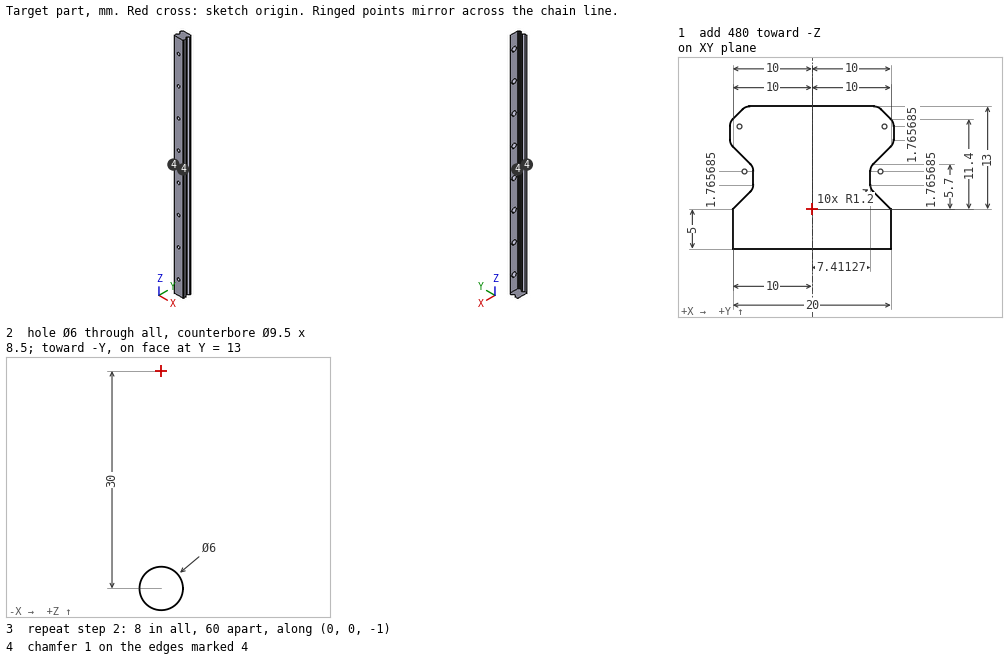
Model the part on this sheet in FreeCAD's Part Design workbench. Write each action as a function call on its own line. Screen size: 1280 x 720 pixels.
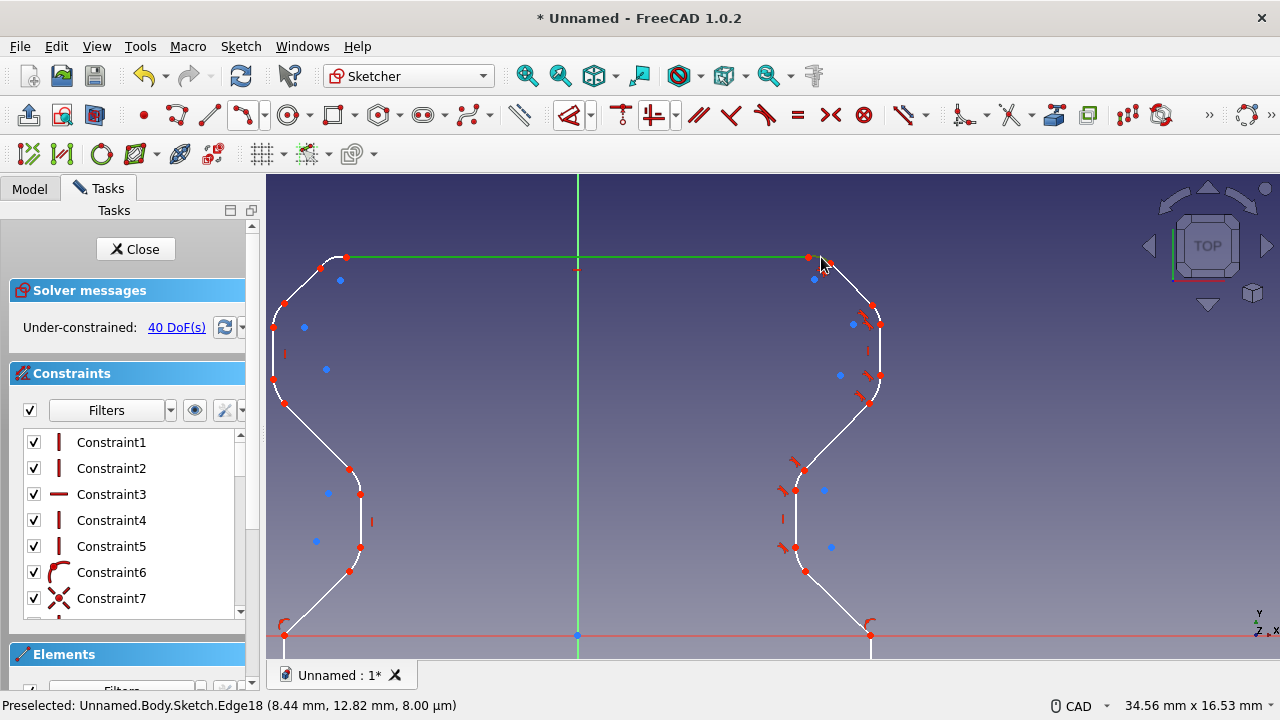
key(t)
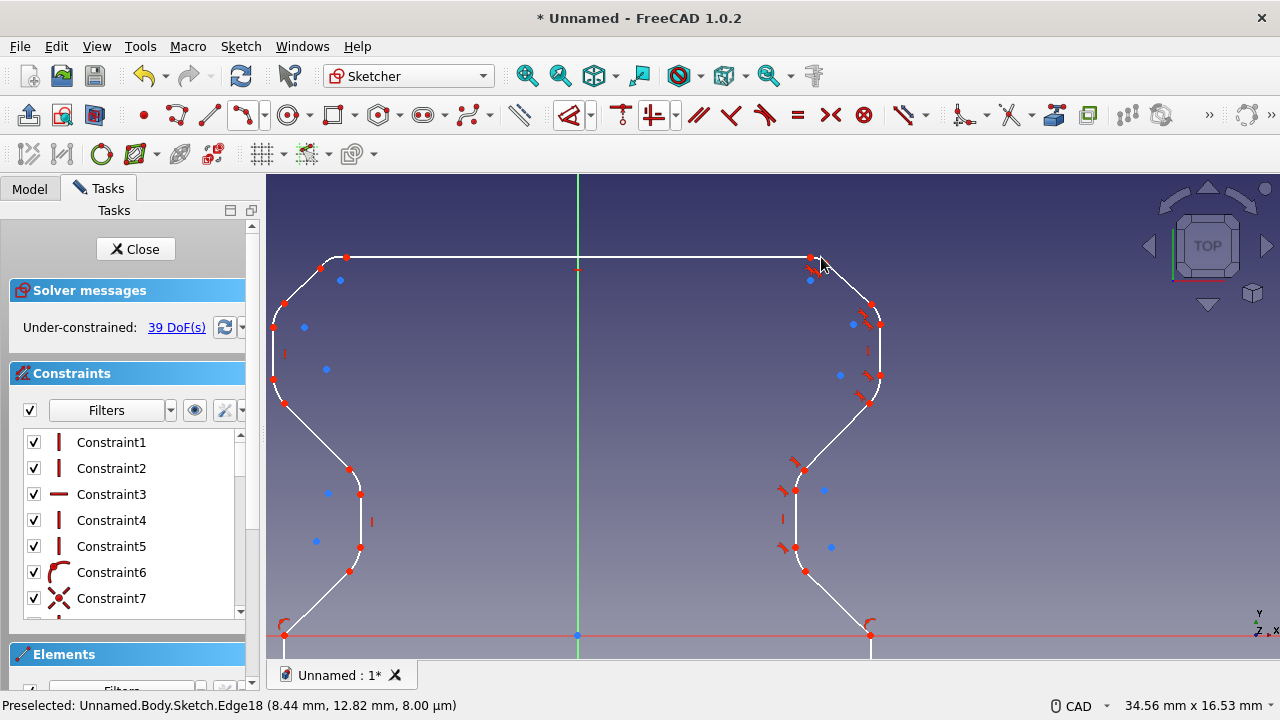
click(671, 257)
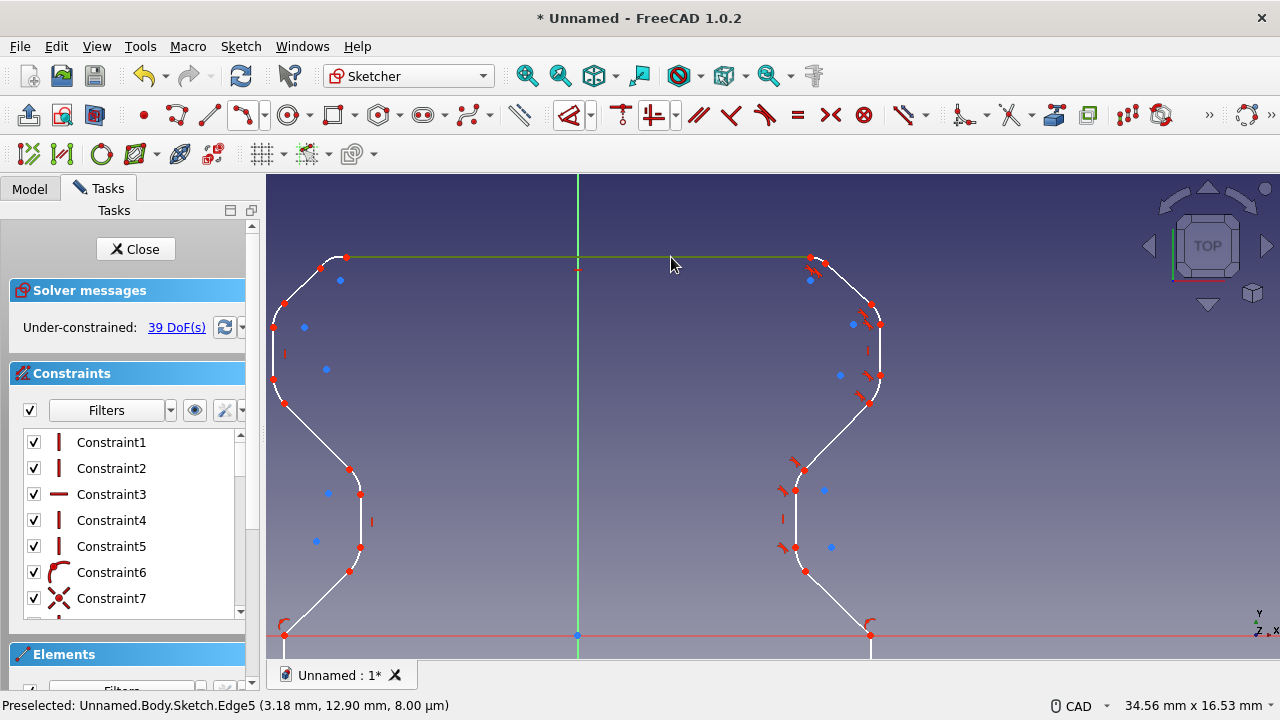
click(332, 258)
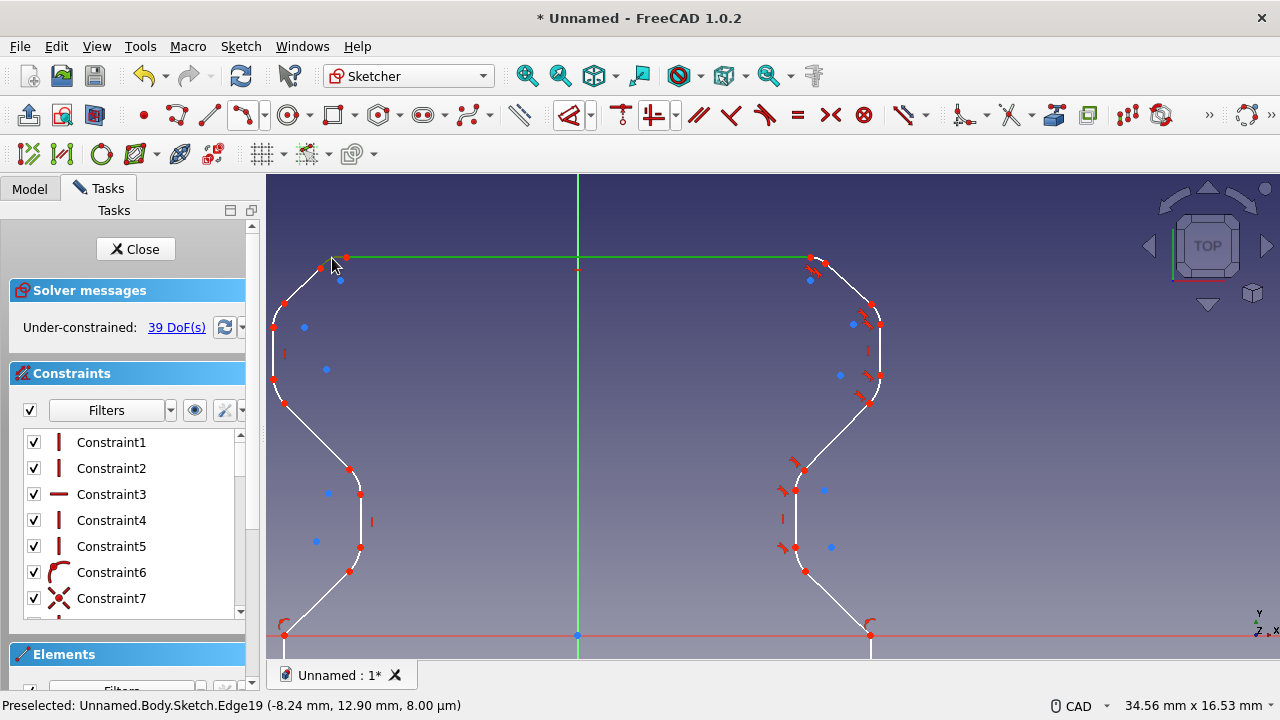
key(t)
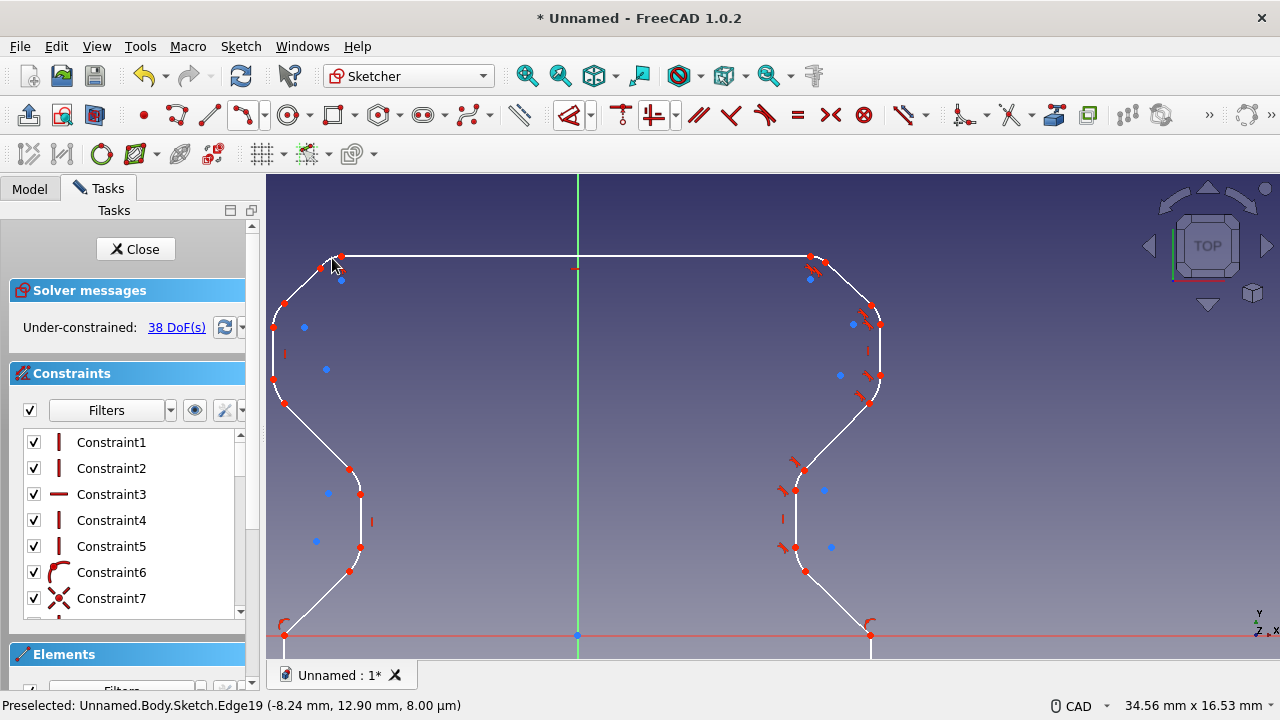
click(310, 279)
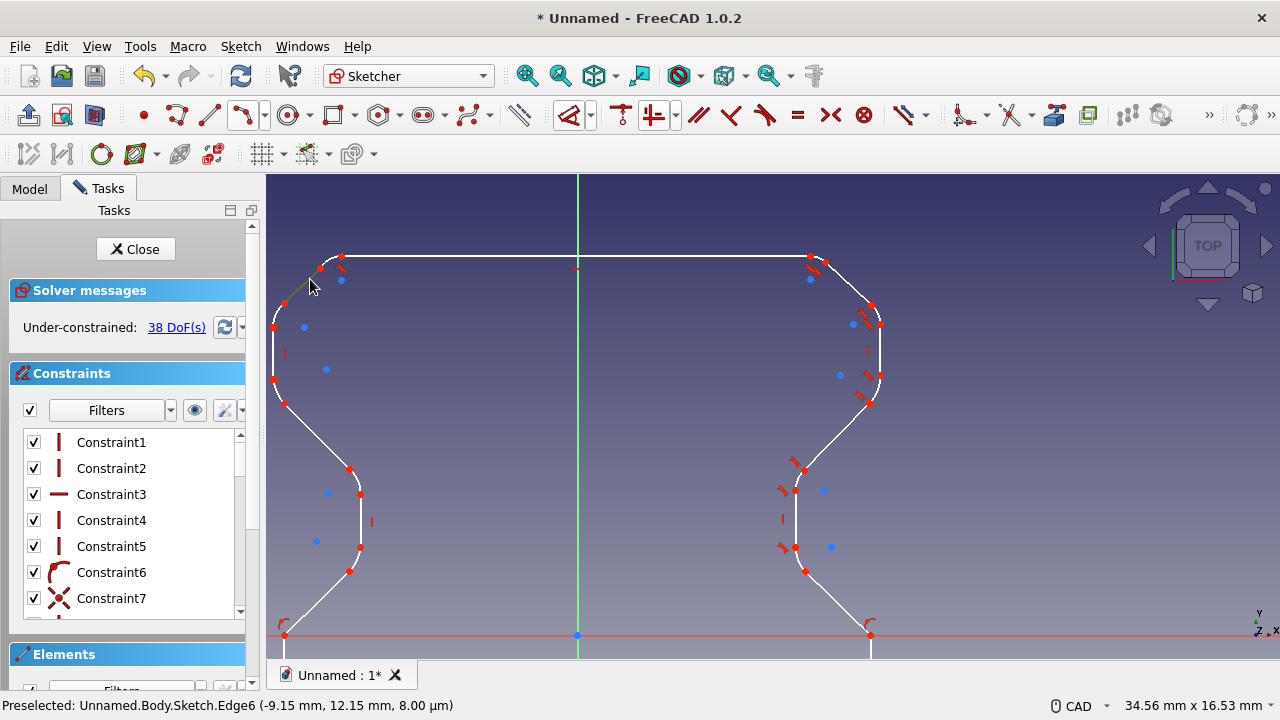
click(329, 259)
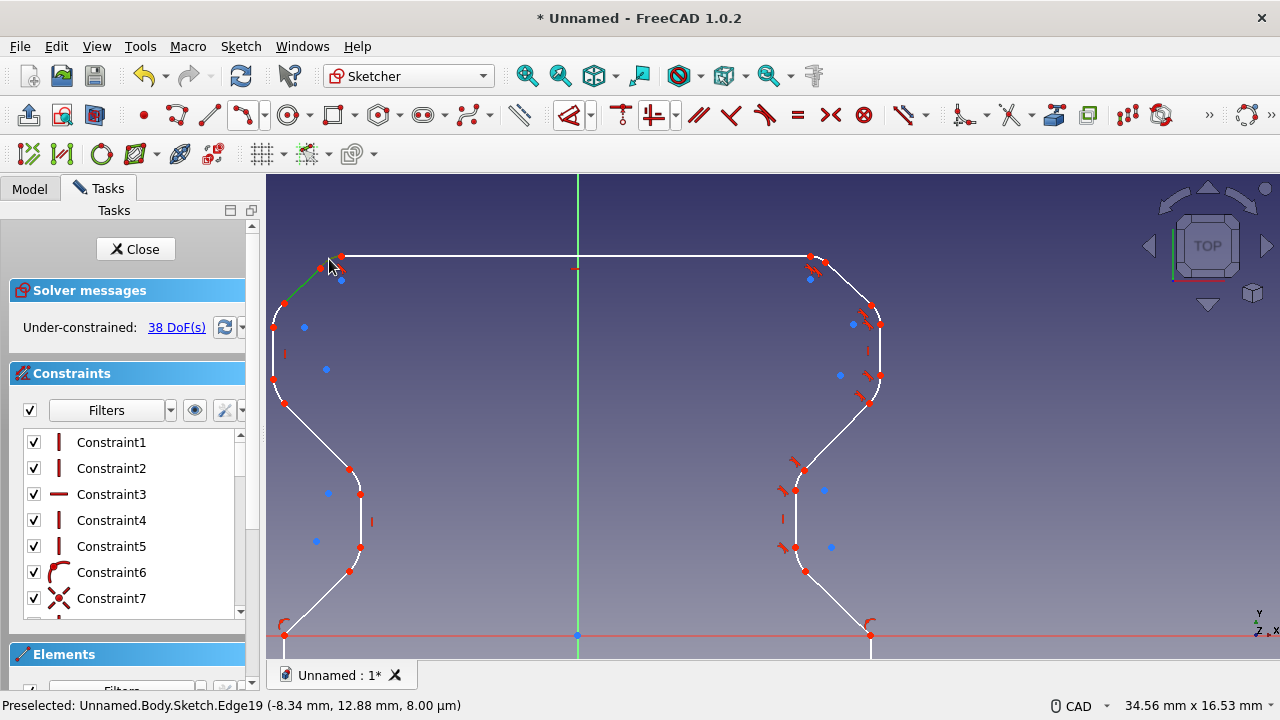
key(t)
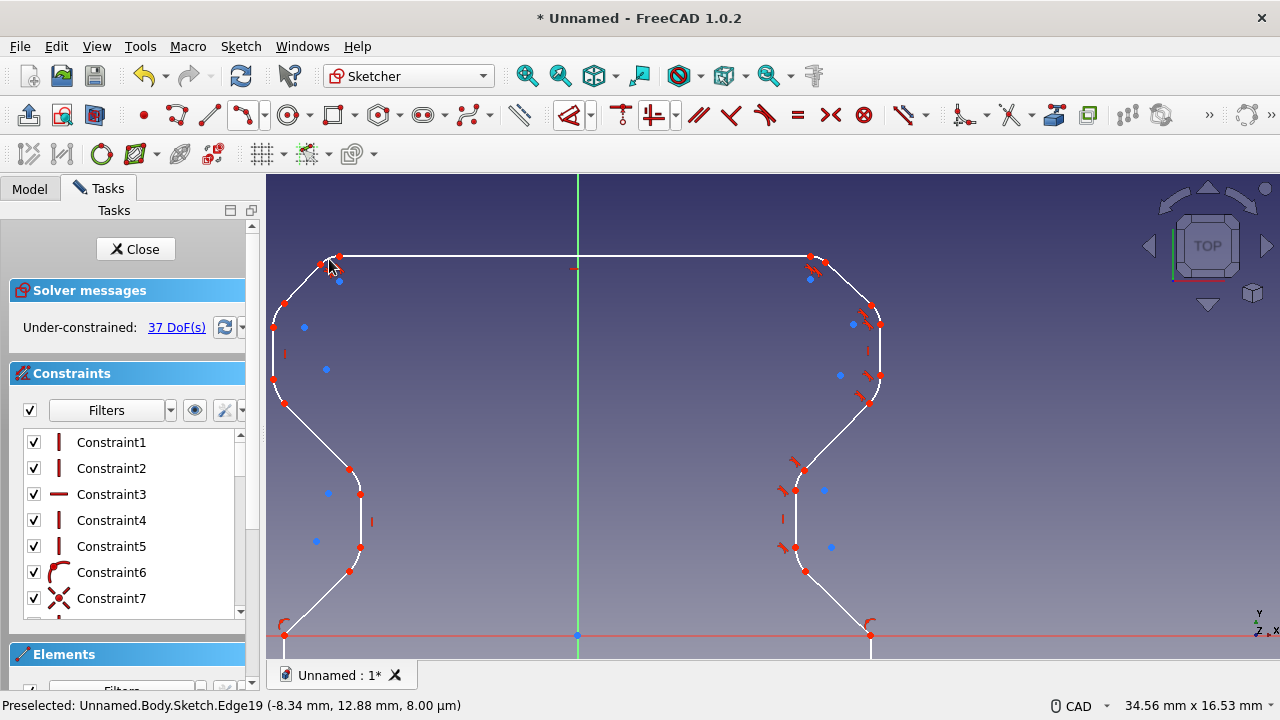
click(310, 276)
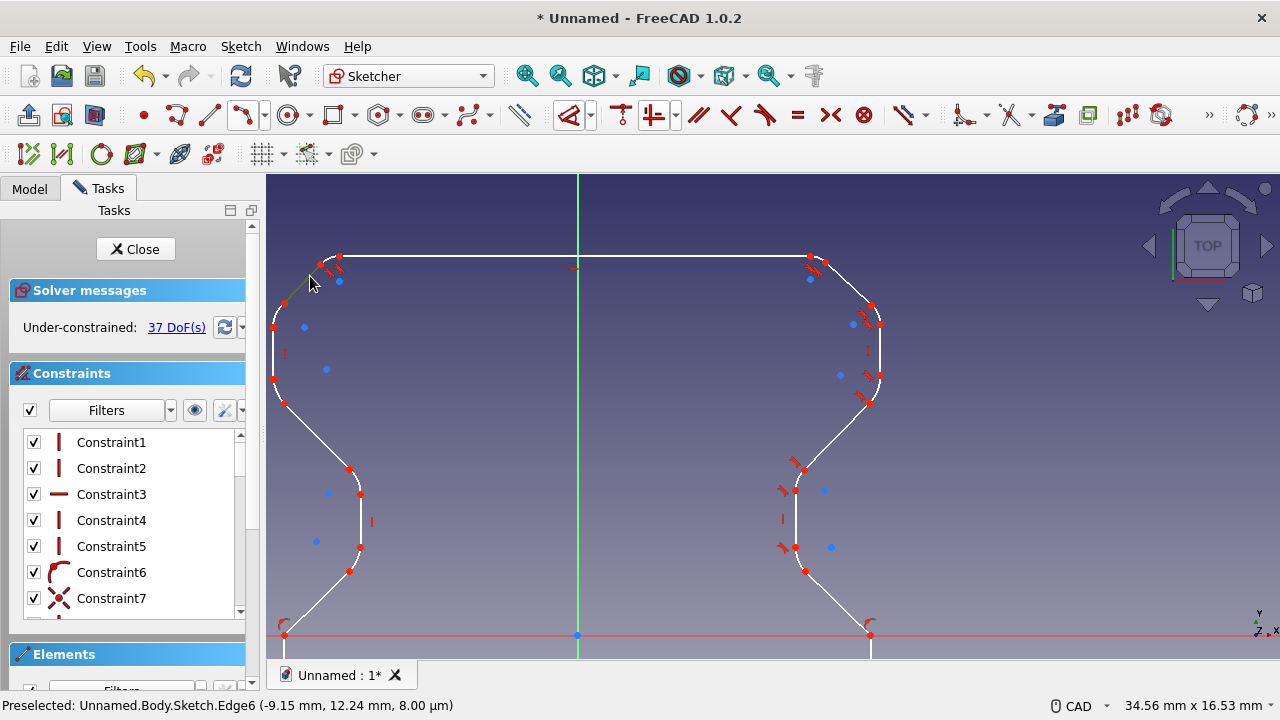
scroll(859, 293, down, 3)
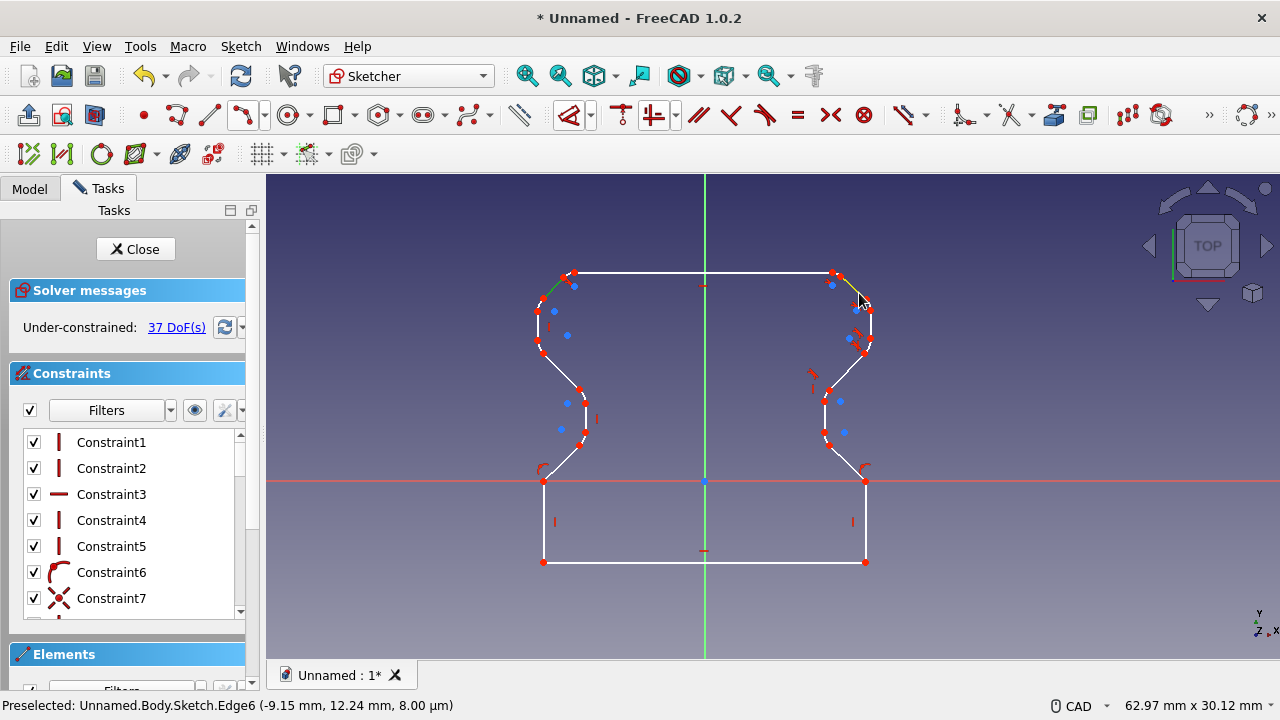
scroll(539, 305, up, 4)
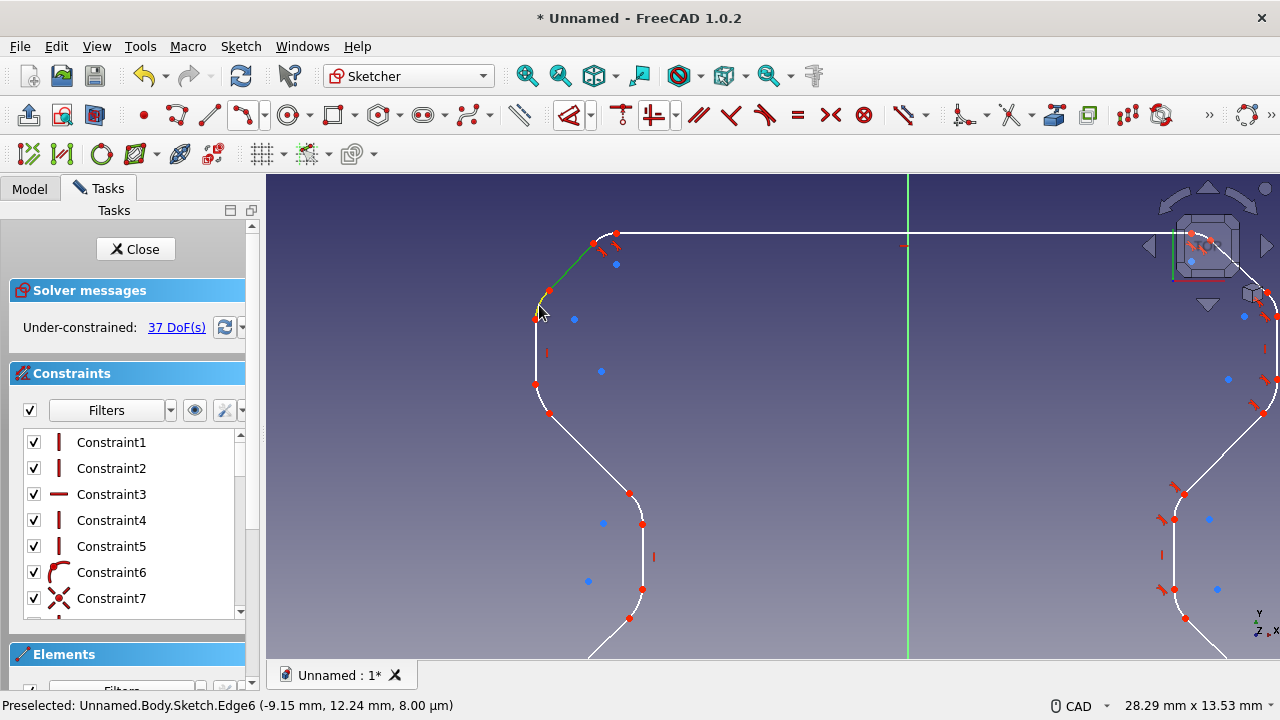
click(539, 304)